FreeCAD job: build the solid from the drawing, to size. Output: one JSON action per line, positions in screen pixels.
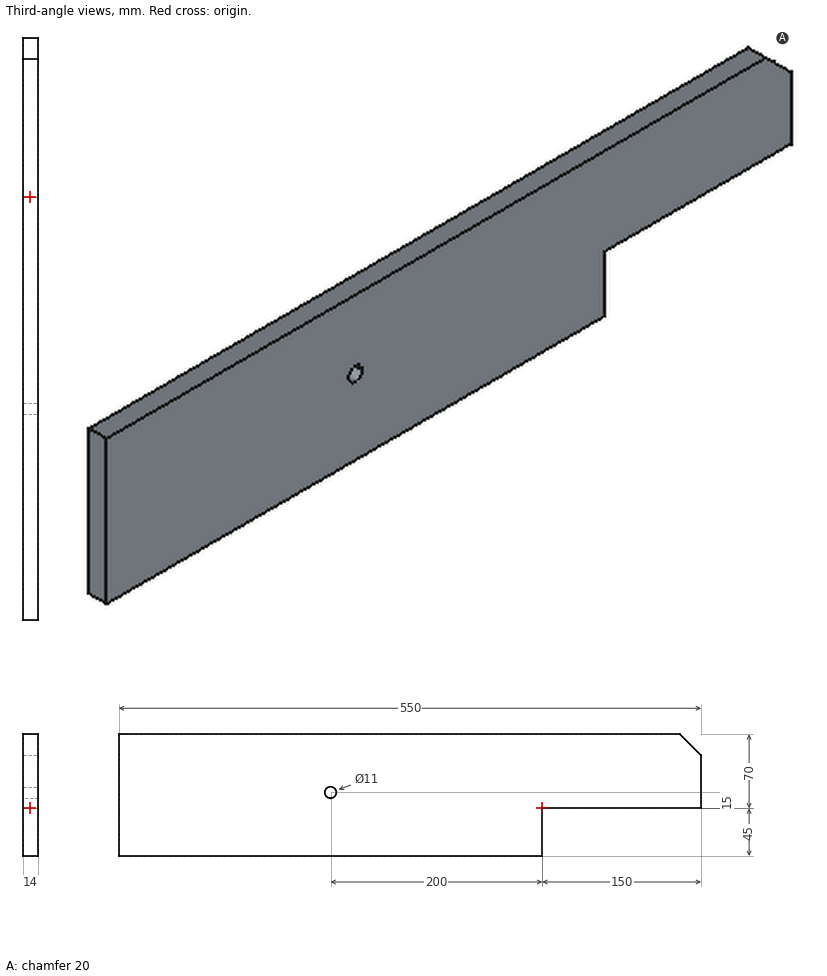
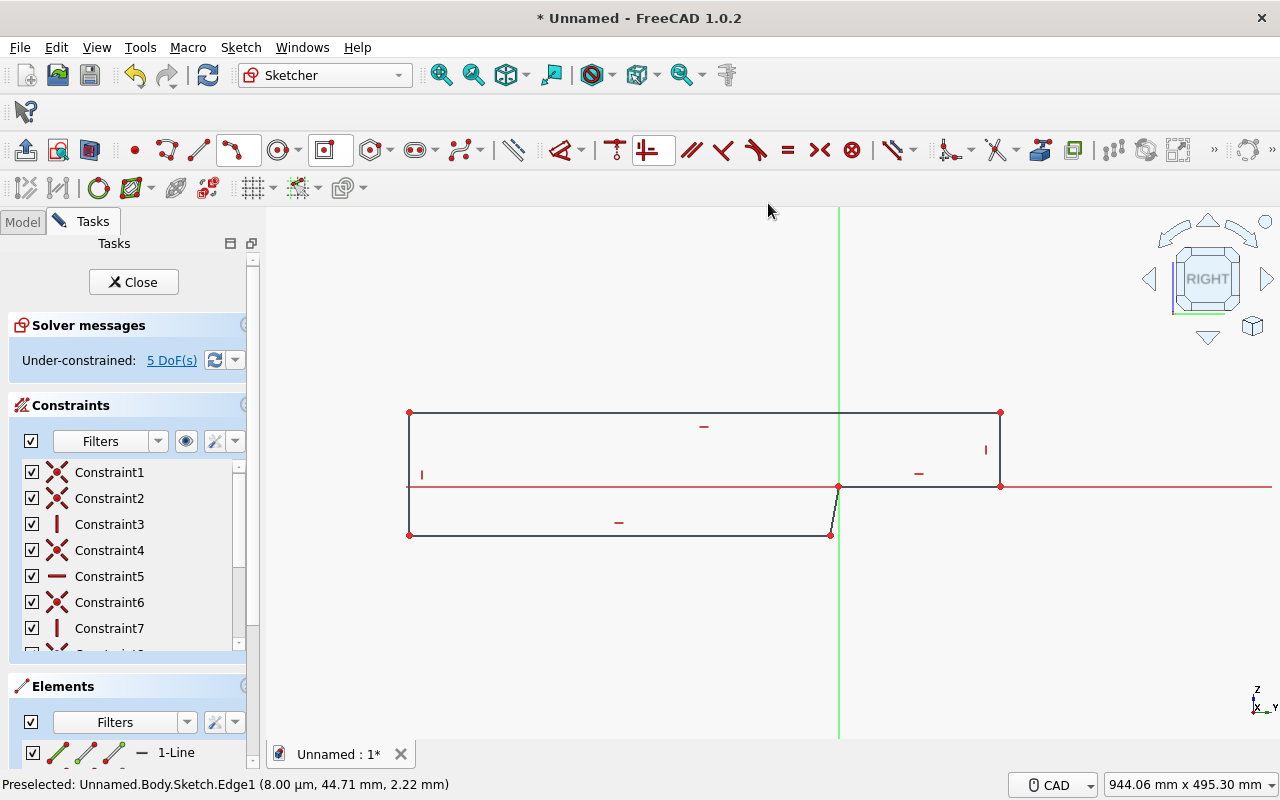
{"action": "left_click", "coordinate": [836, 502]}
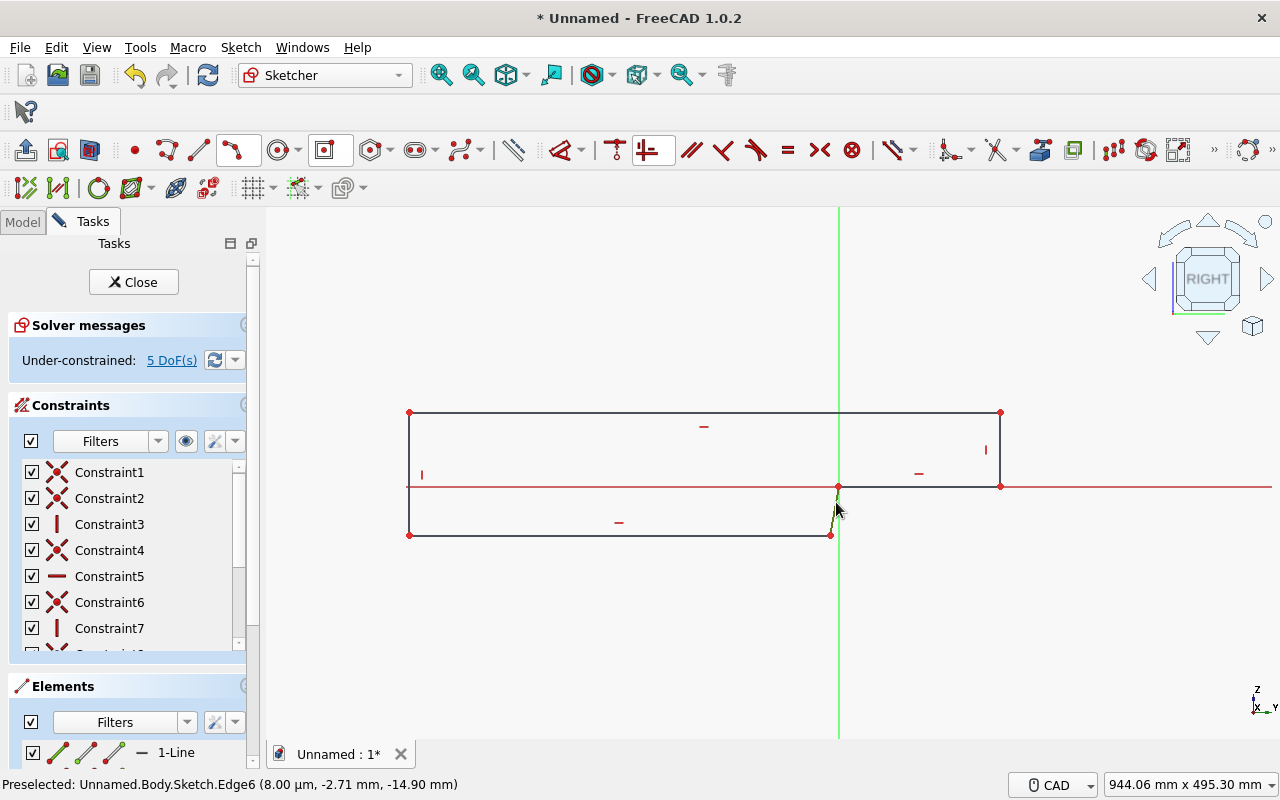
{"action": "left_click", "coordinate": [670, 150]}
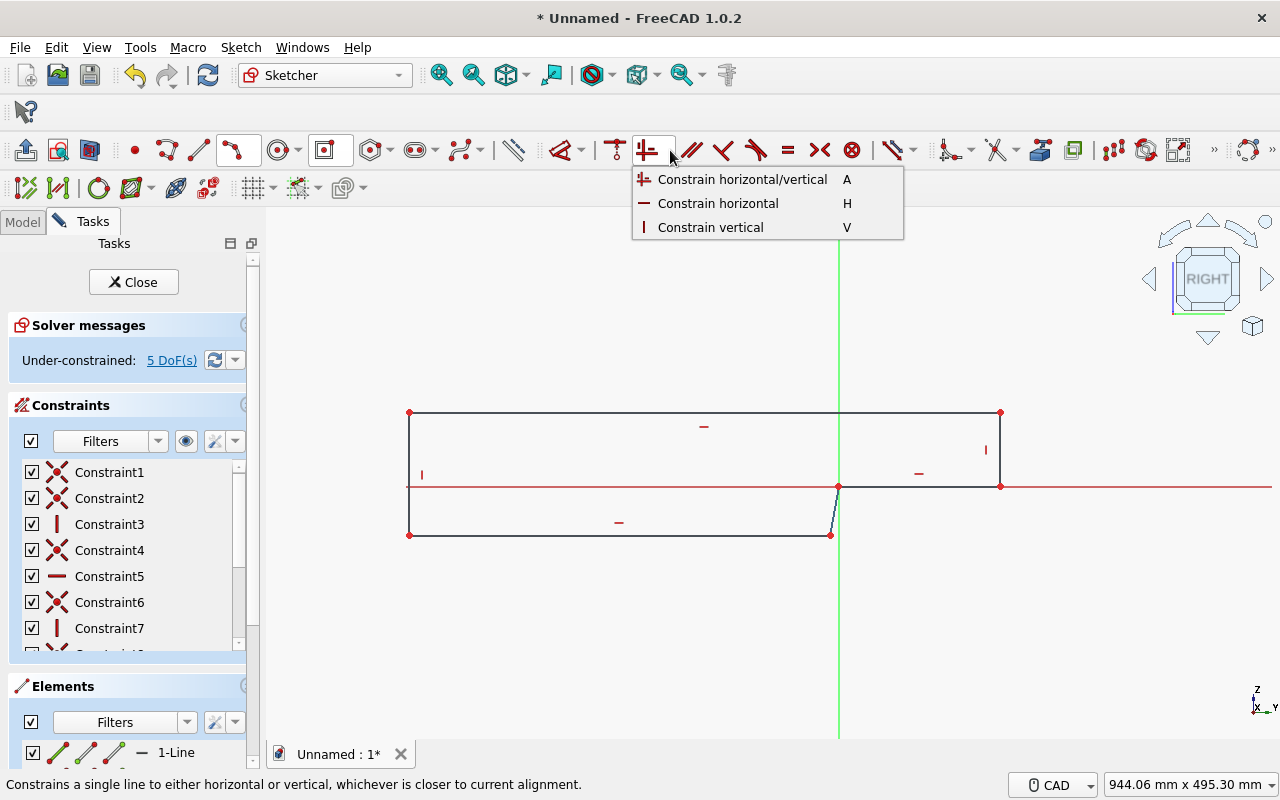
{"action": "left_click", "coordinate": [768, 227]}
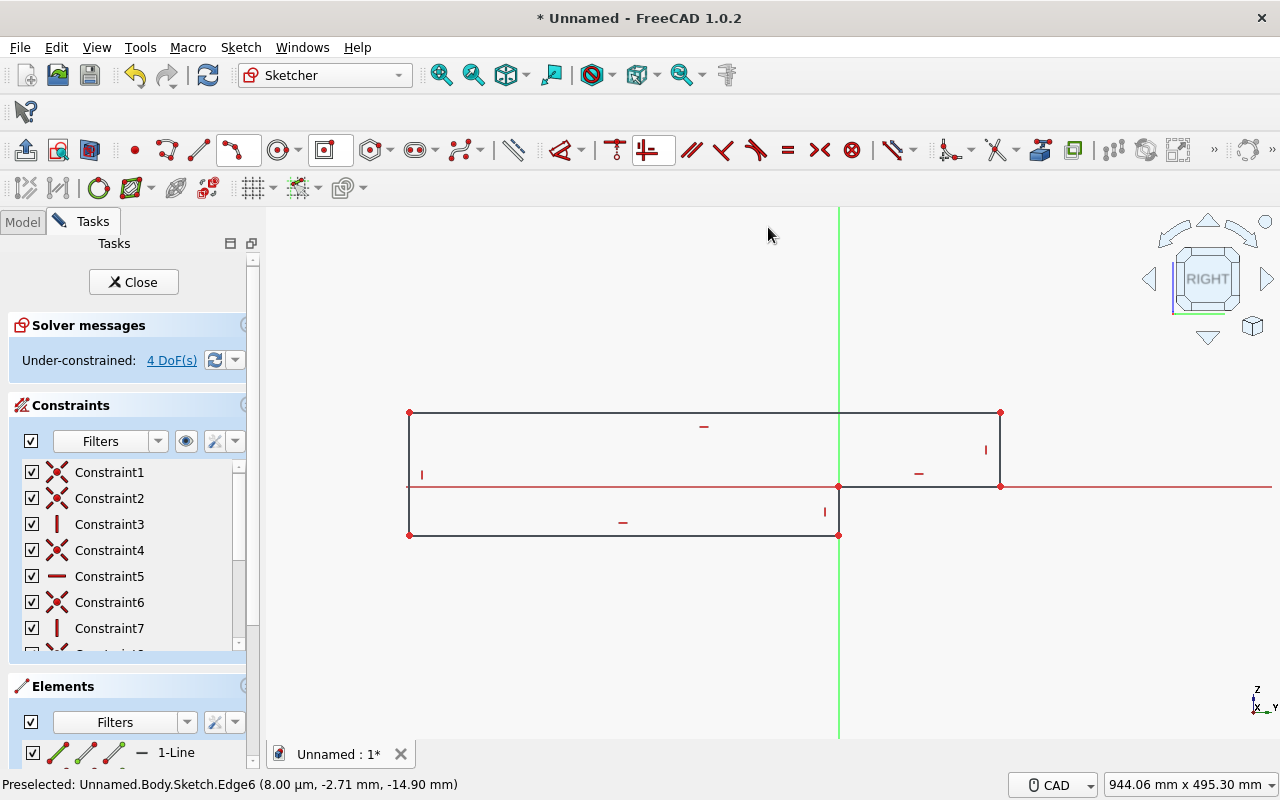
{"action": "left_click", "coordinate": [1000, 465]}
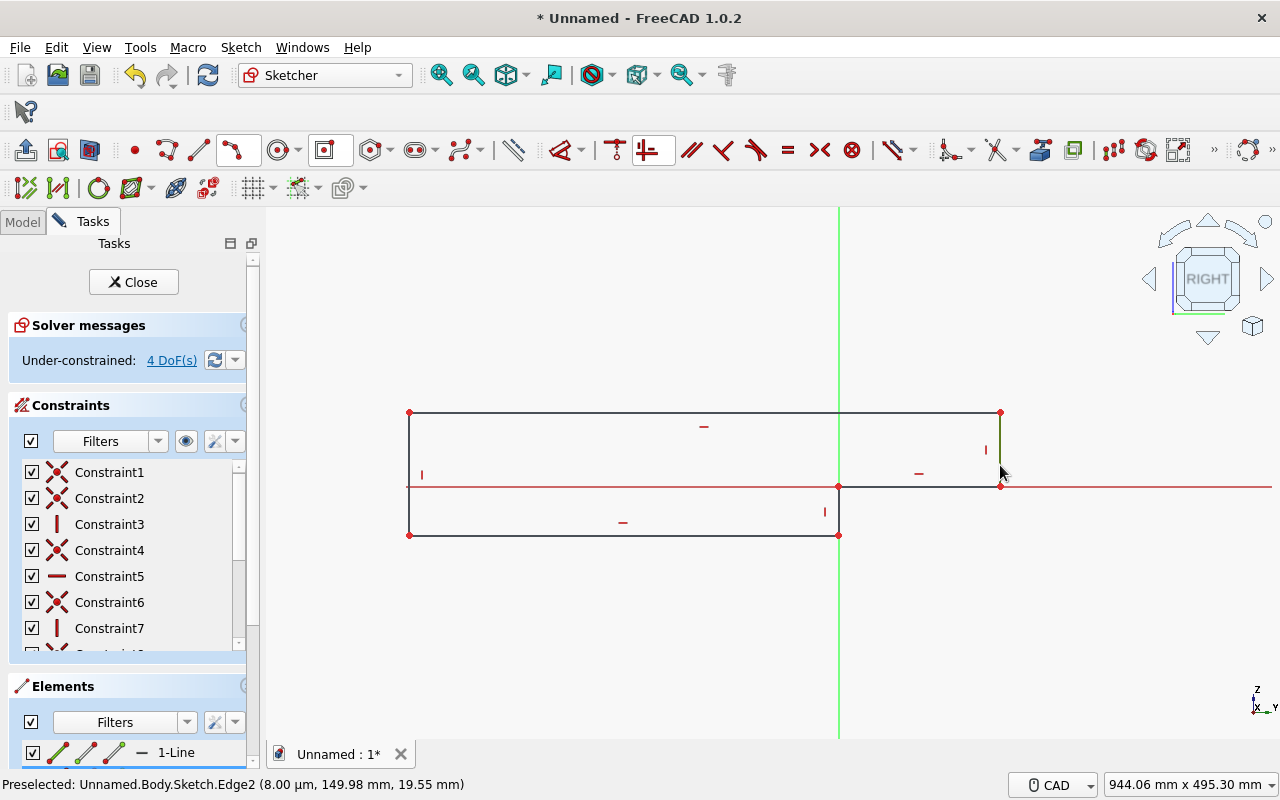
{"action": "key", "text": "i"}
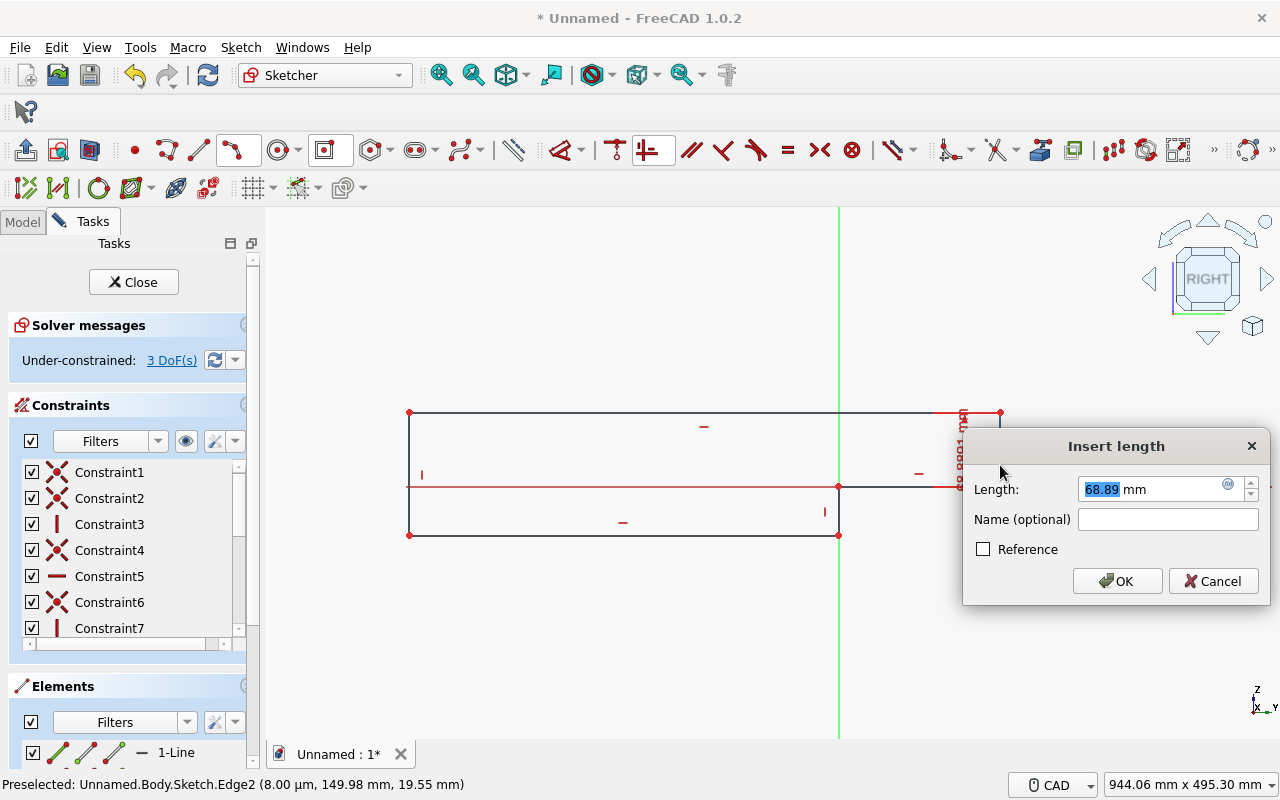
{"action": "type", "text": "70"}
{"action": "key", "text": "Return"}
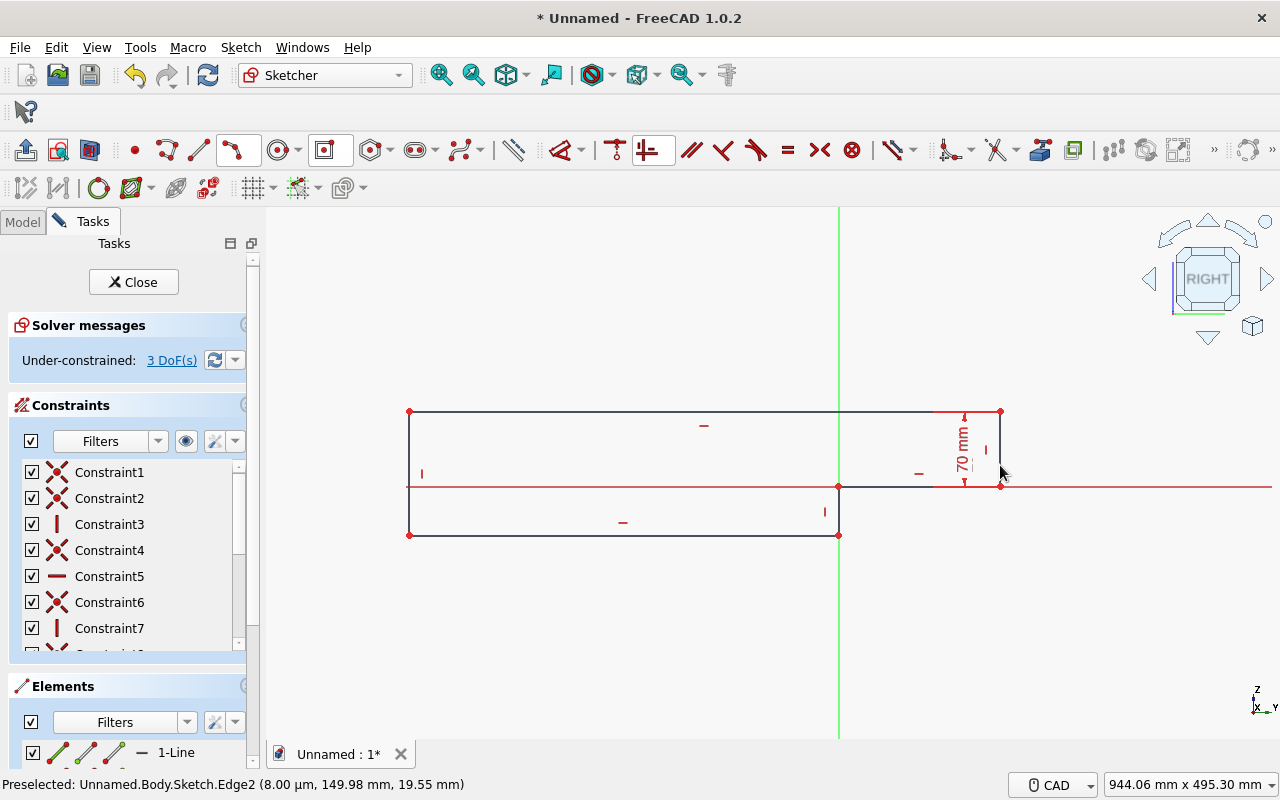
{"action": "left_click", "coordinate": [839, 521]}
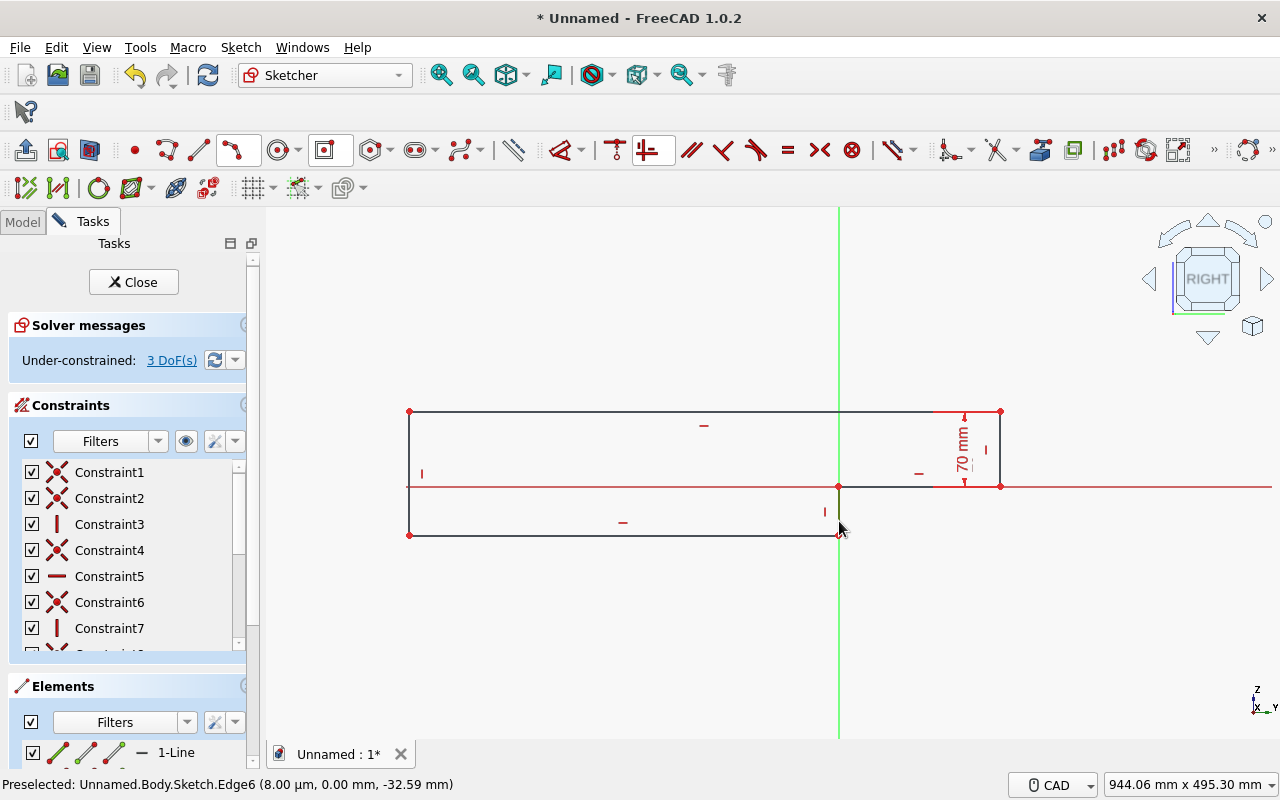
{"action": "left_click", "coordinate": [584, 150]}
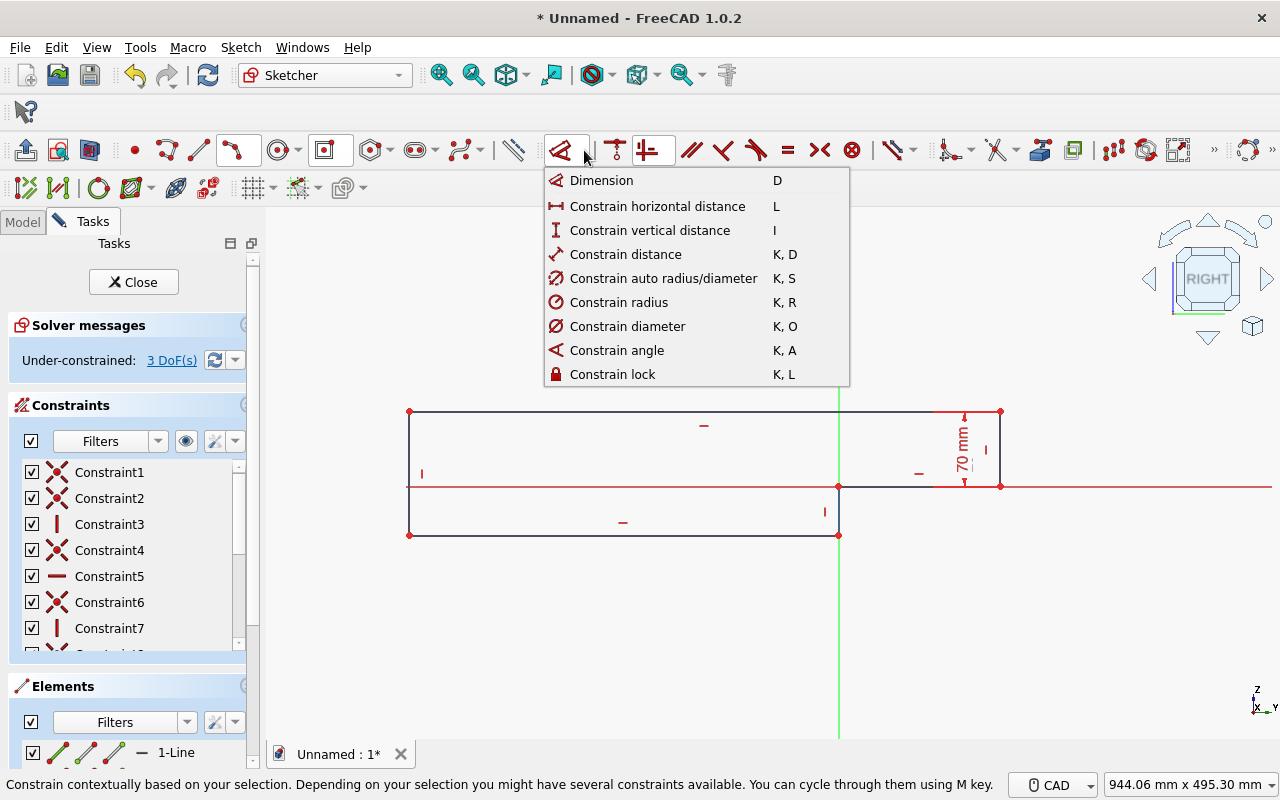
{"action": "left_click", "coordinate": [697, 230]}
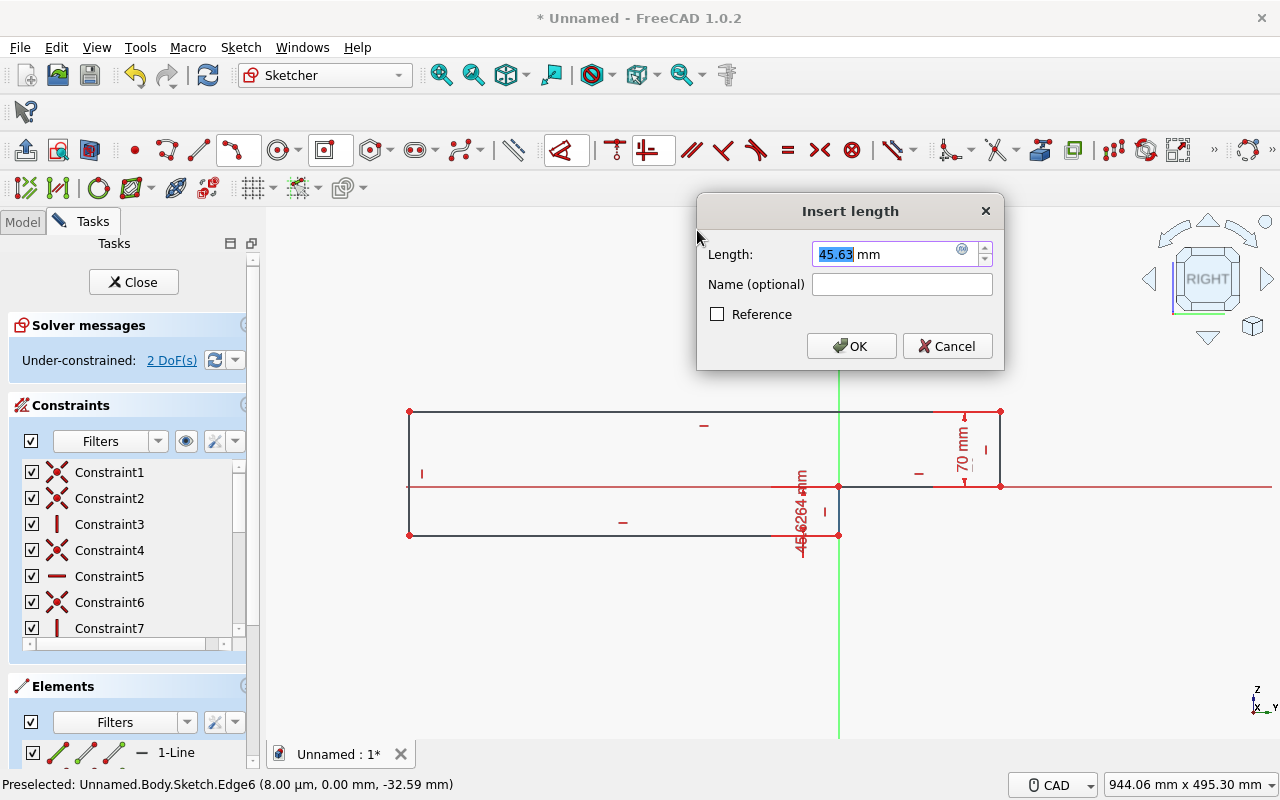
{"action": "type", "text": "45"}
{"action": "key", "text": "Return"}